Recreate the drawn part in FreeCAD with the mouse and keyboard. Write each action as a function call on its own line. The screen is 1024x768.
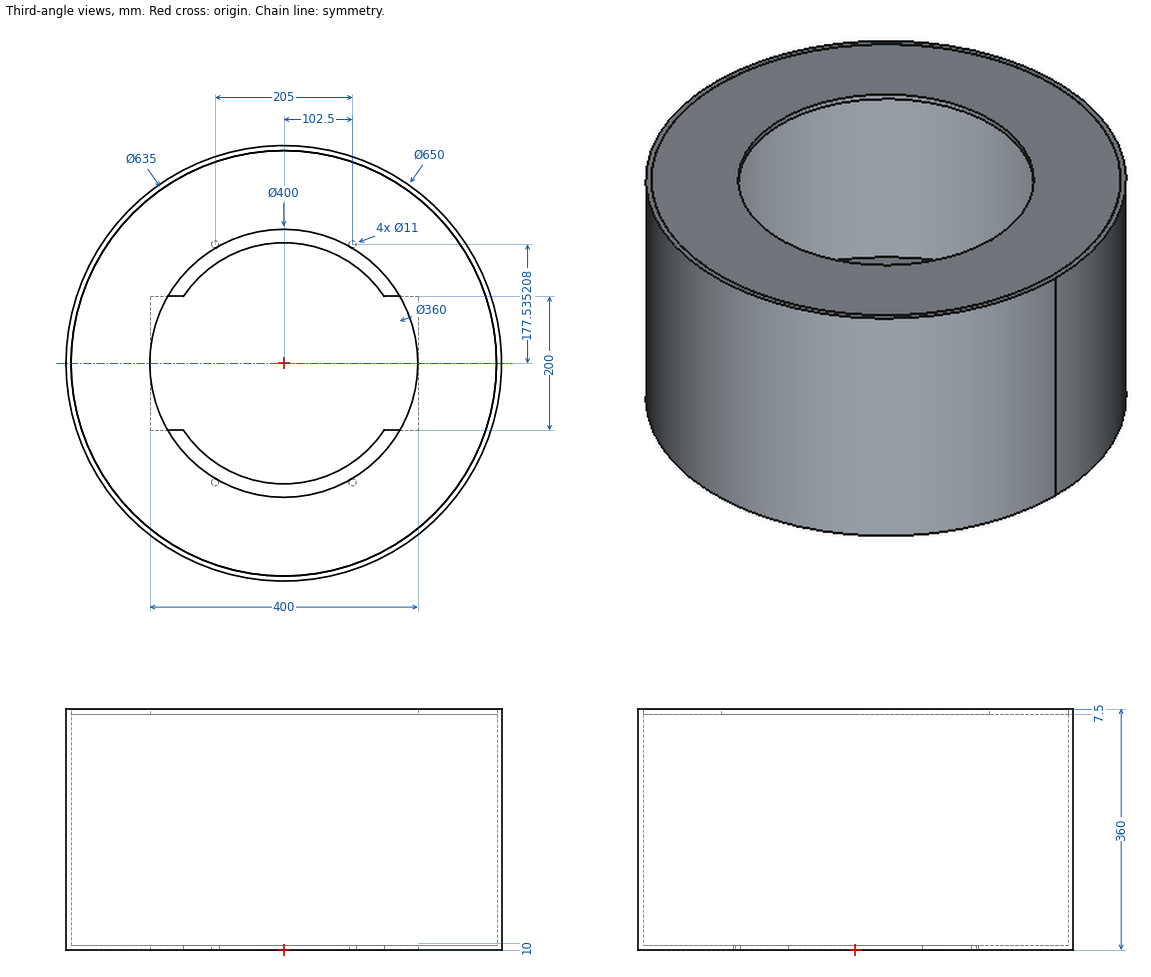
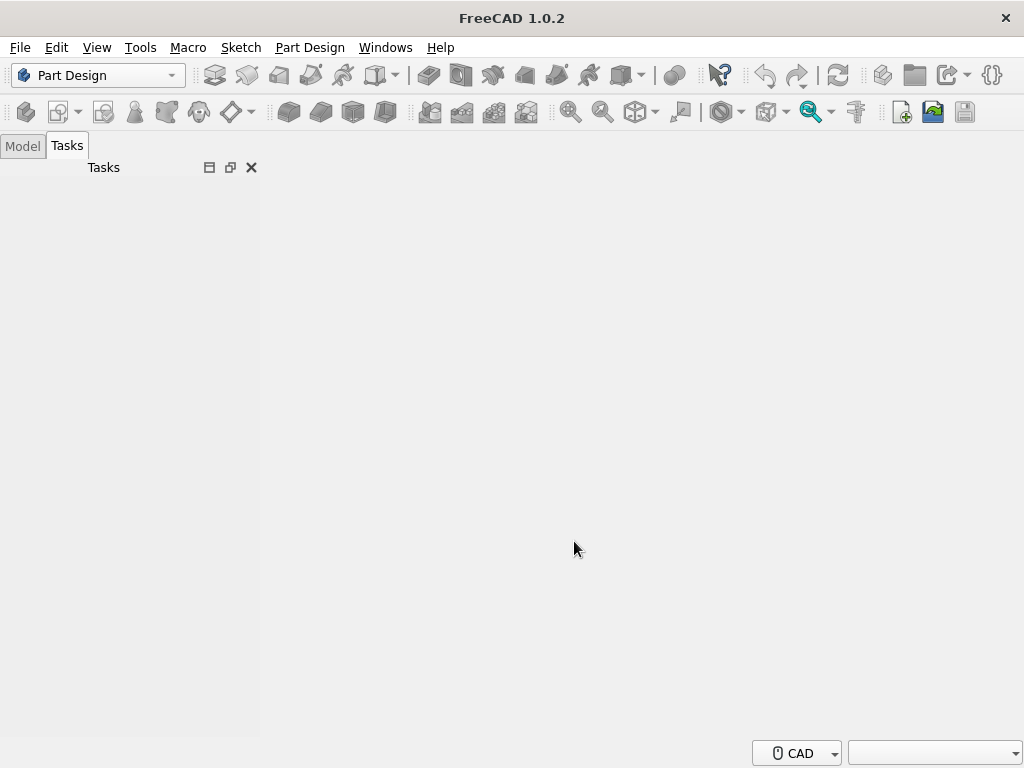
click(902, 112)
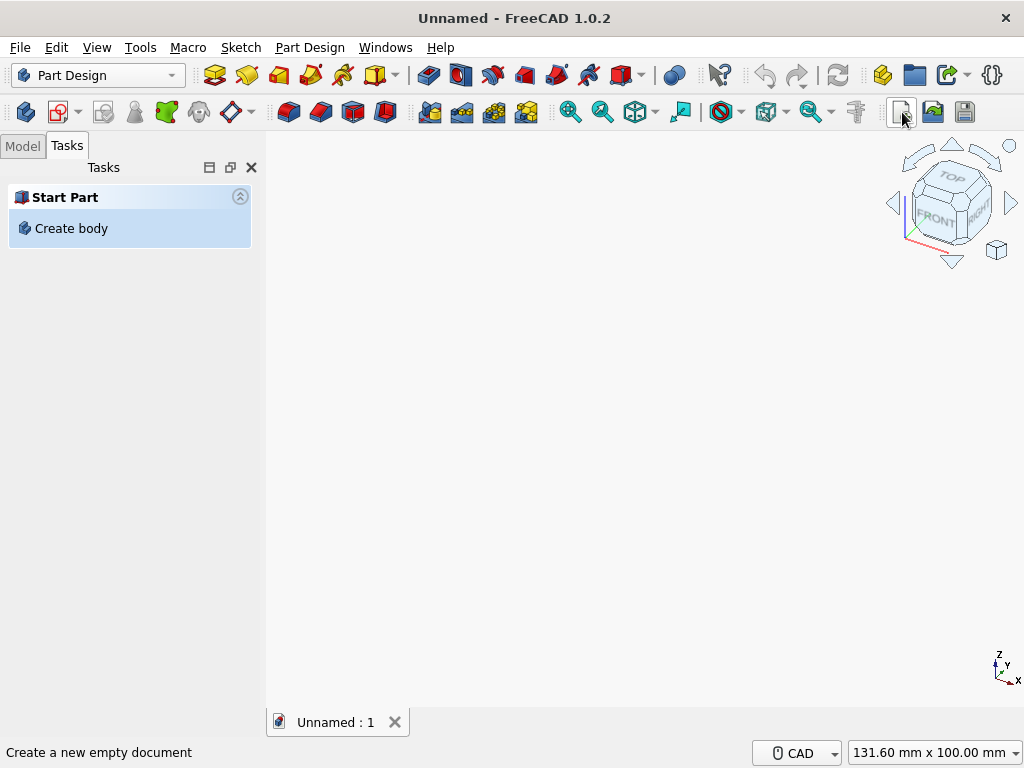
click(58, 112)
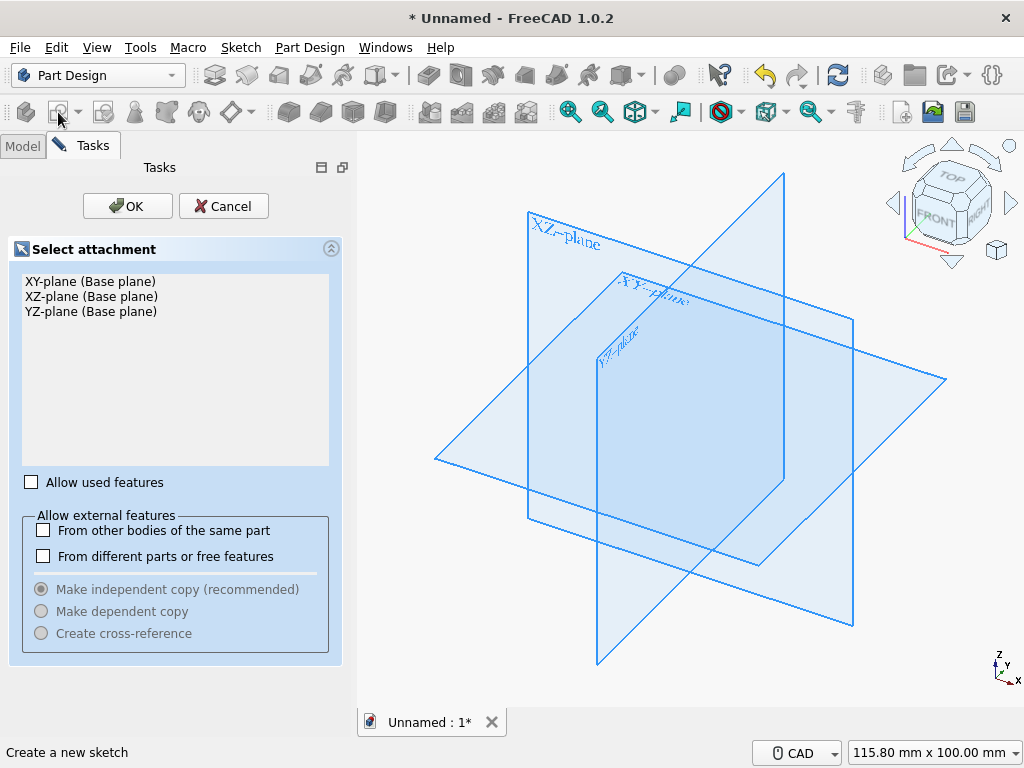
click(82, 282)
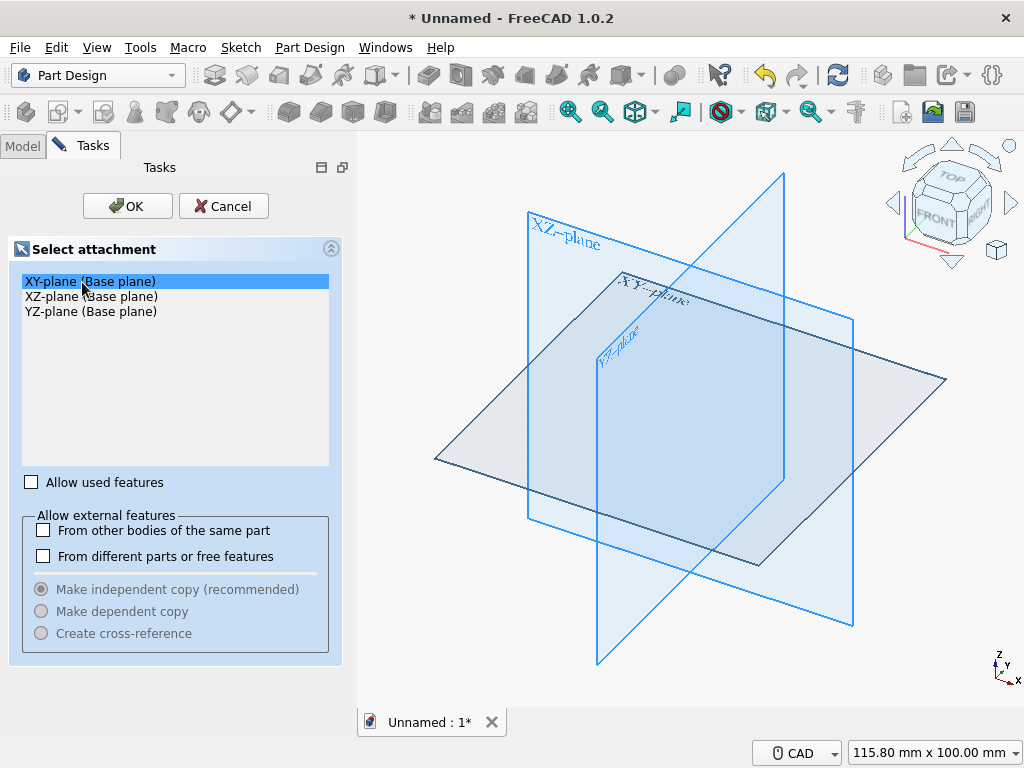
click(128, 206)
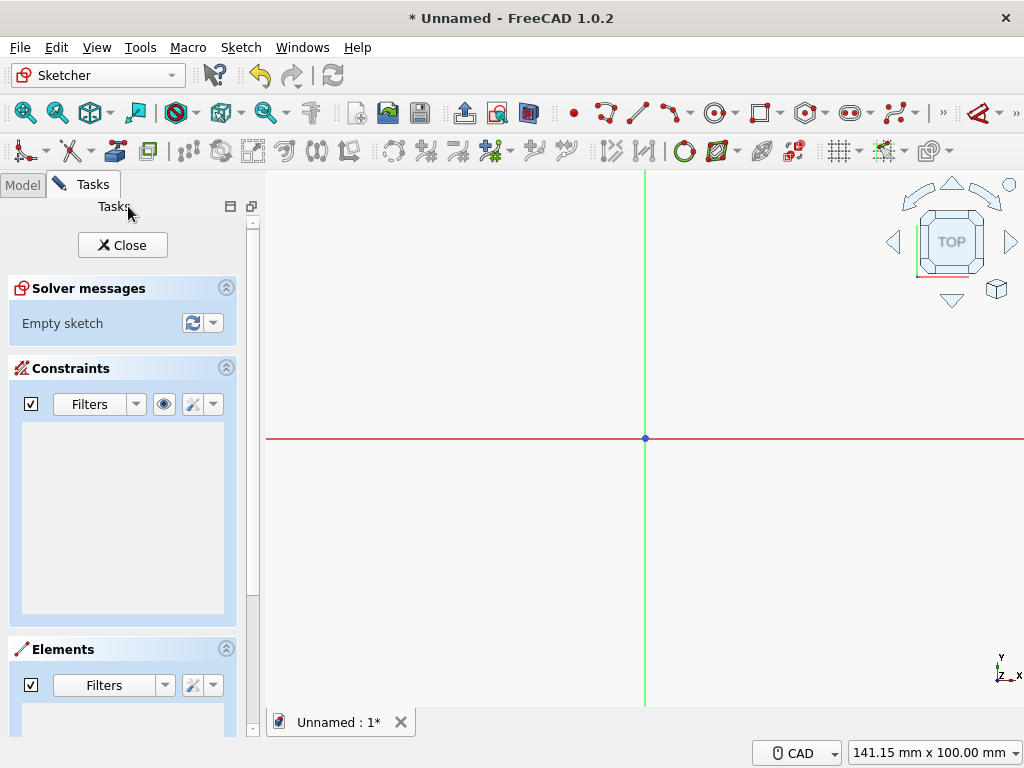
scroll(570, 438, down, 12)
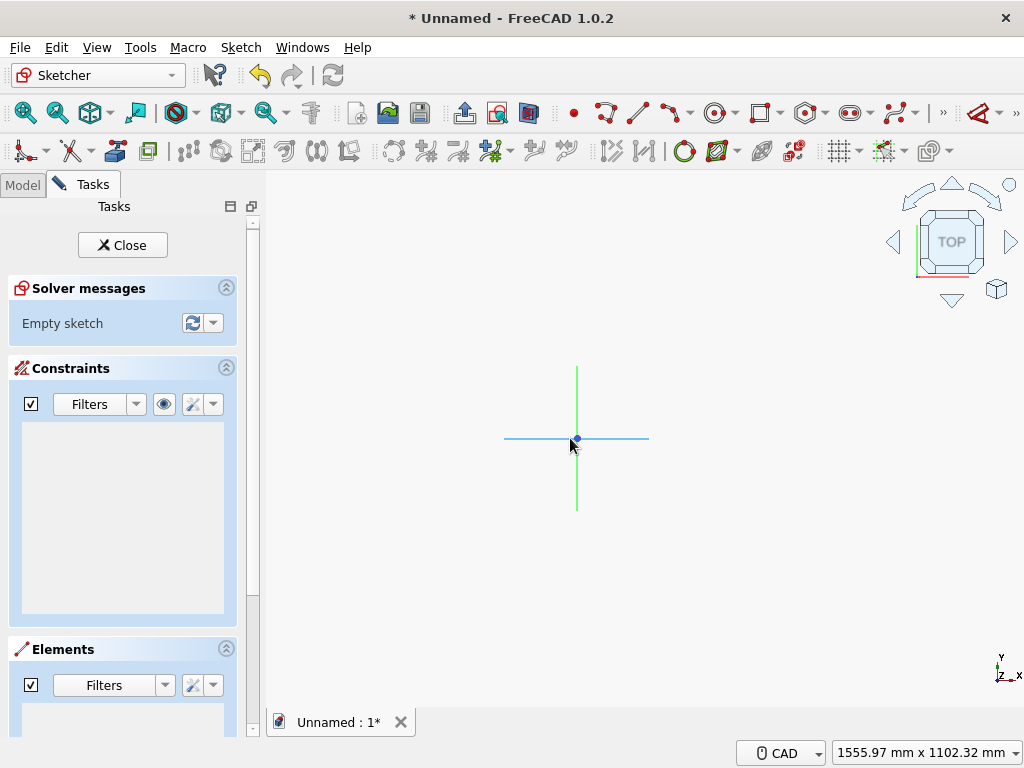
click(716, 114)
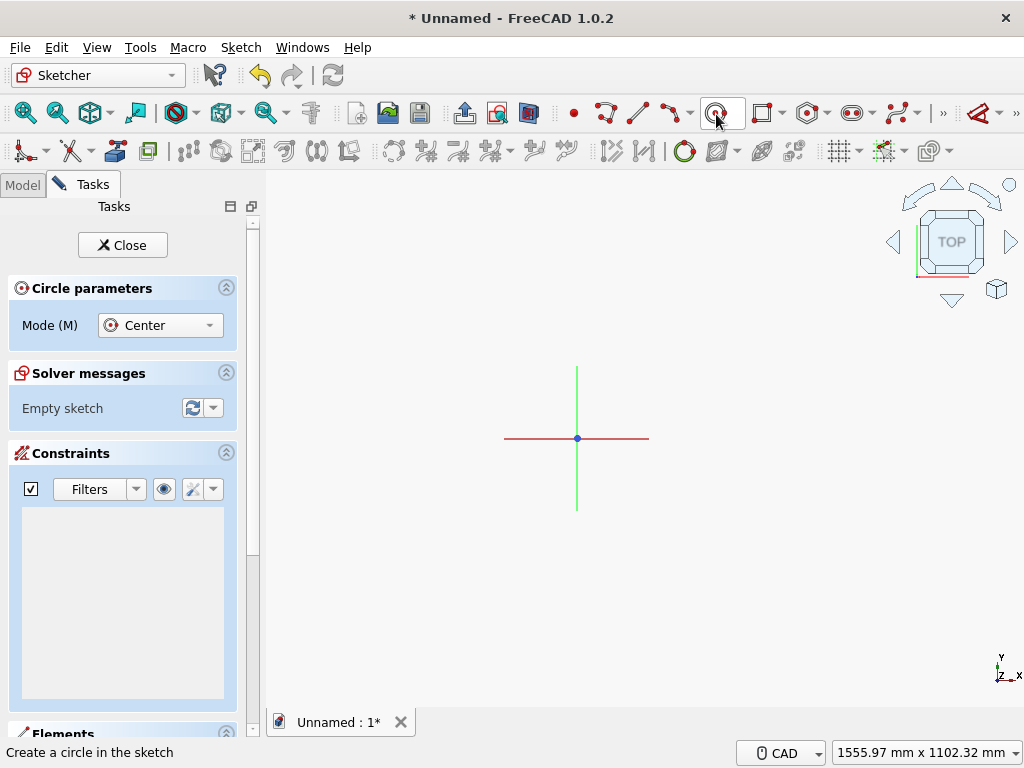
click(577, 438)
click(689, 327)
key(Escape)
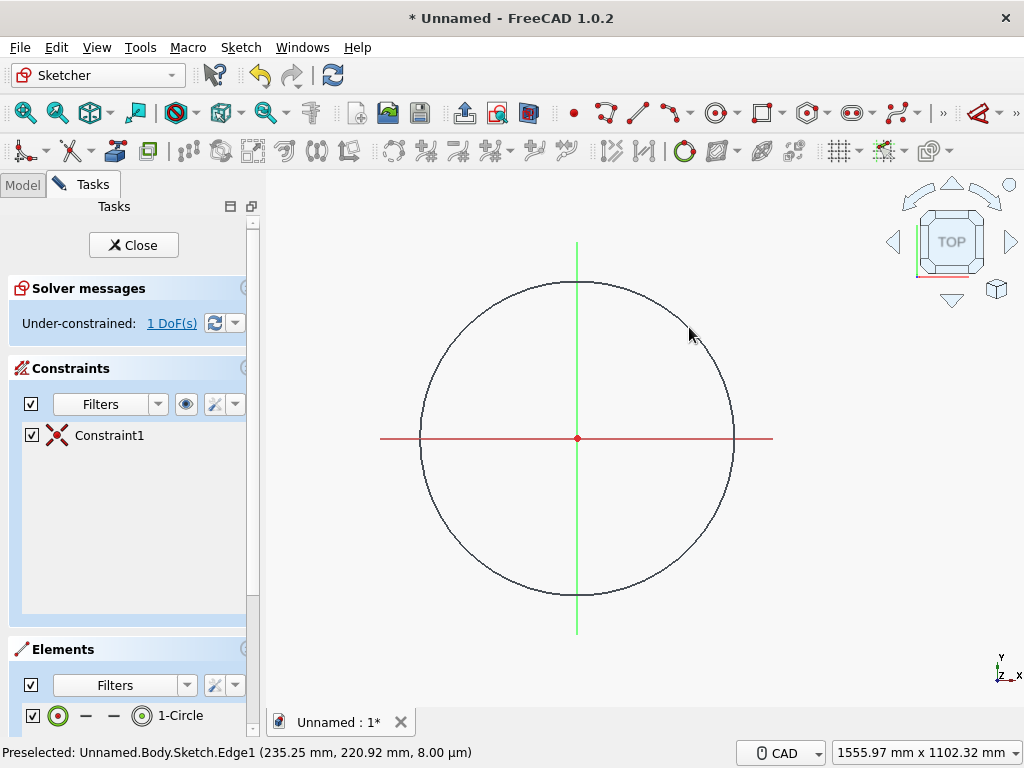
click(978, 114)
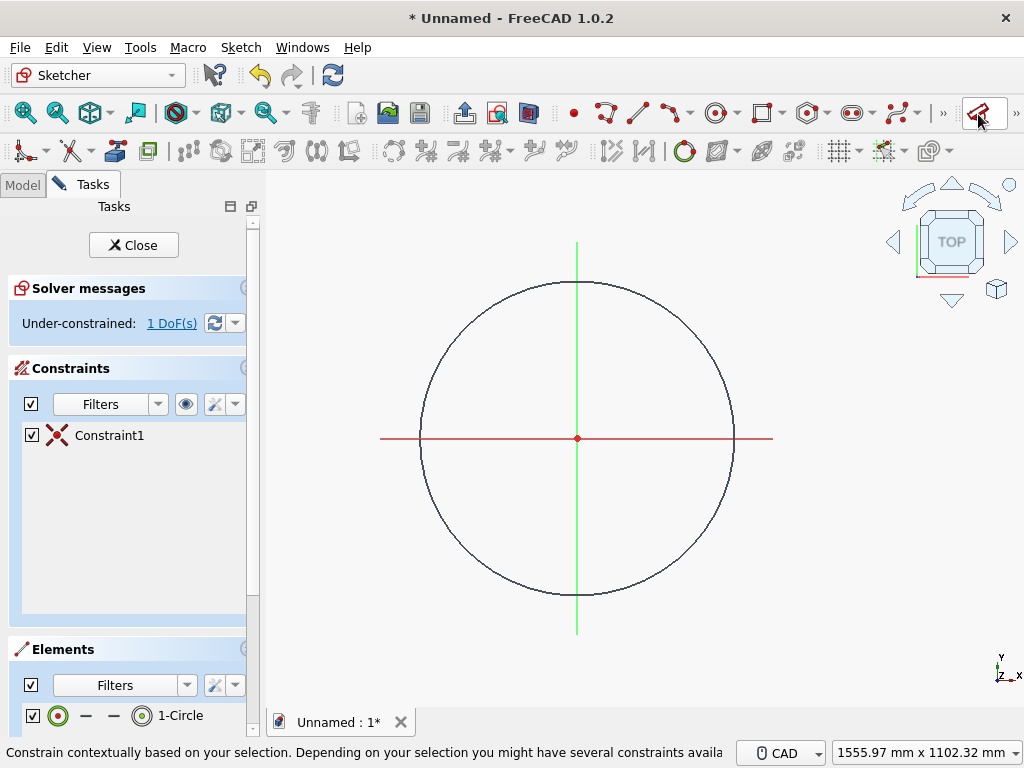
click(688, 327)
click(711, 304)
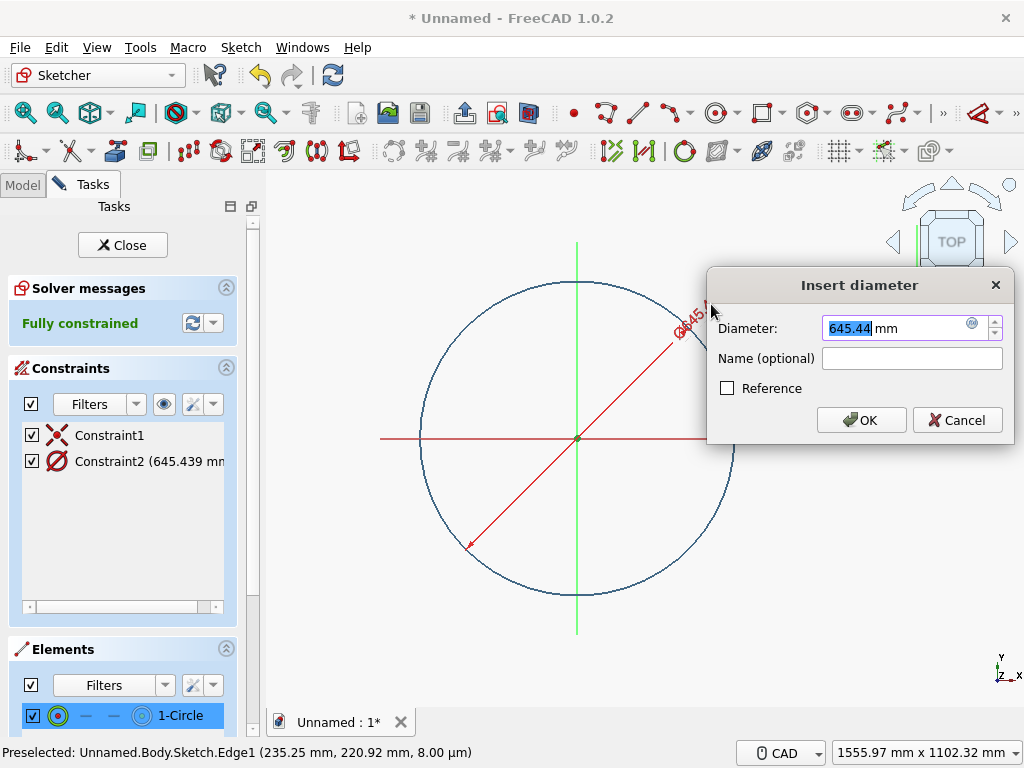
text(650)
key(Return)
key(Escape)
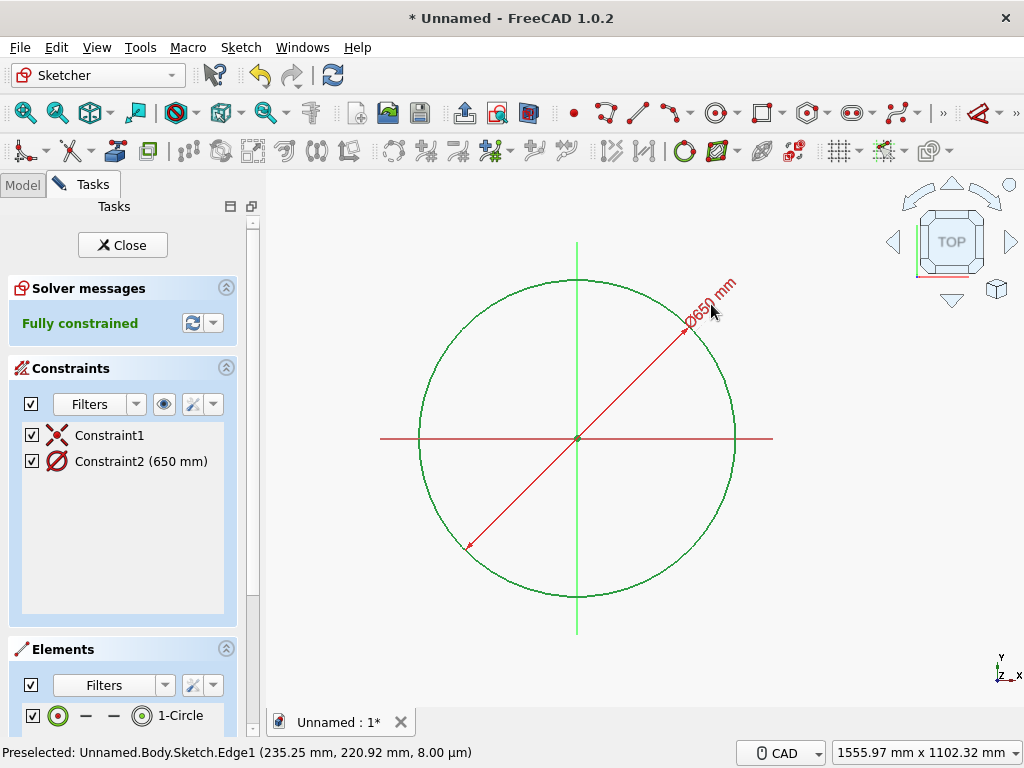
click(123, 245)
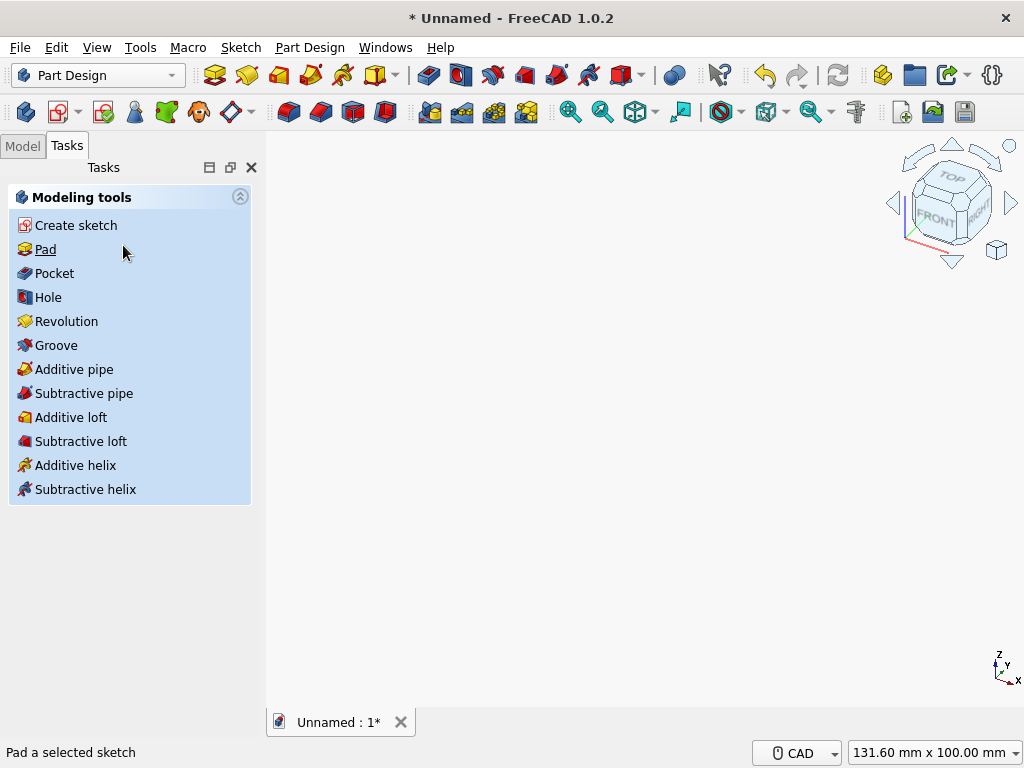
click(216, 76)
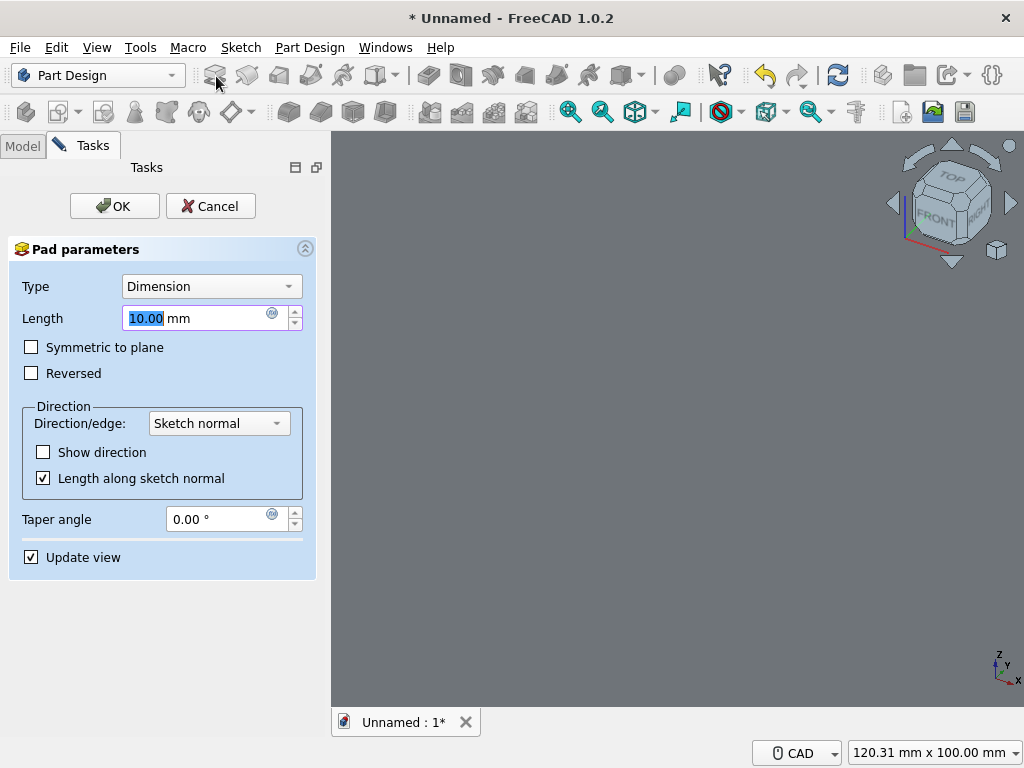
text(360)
key(Tab)